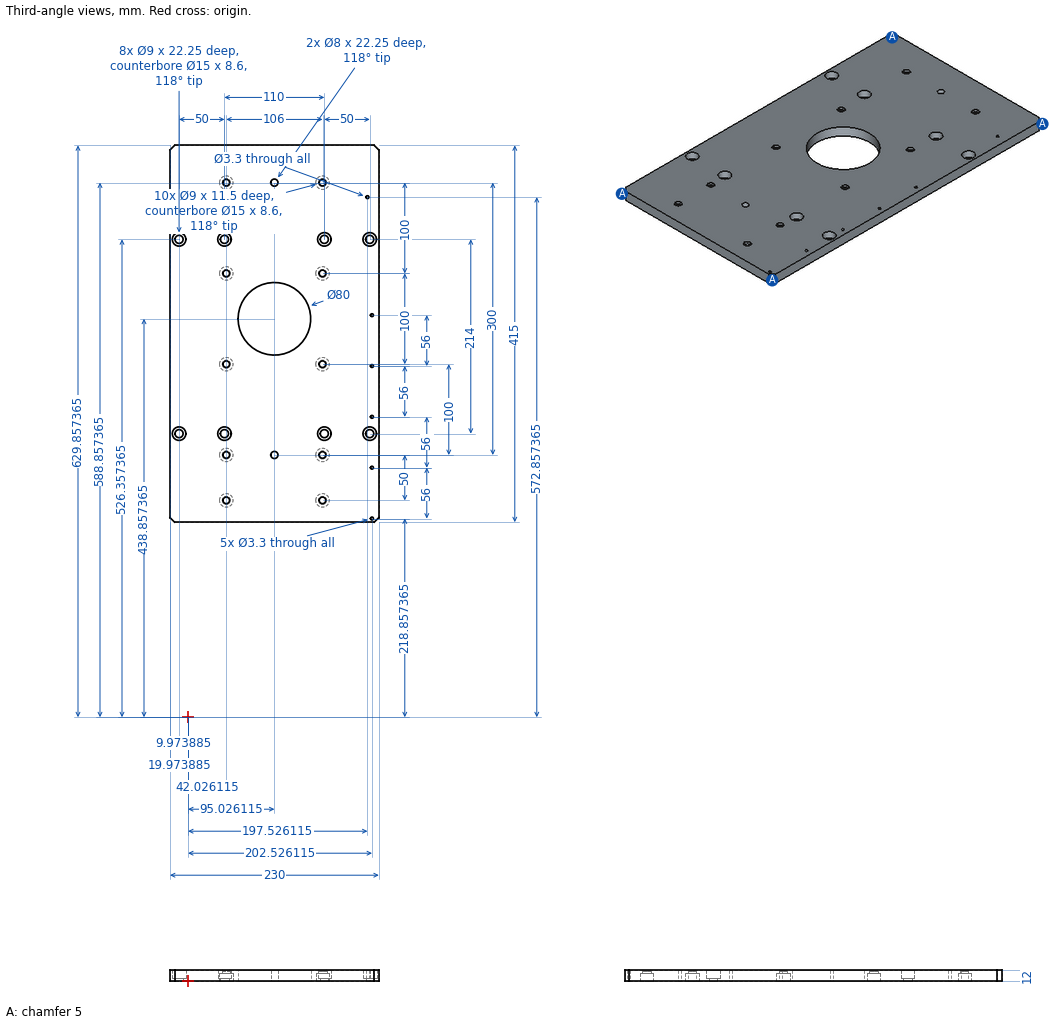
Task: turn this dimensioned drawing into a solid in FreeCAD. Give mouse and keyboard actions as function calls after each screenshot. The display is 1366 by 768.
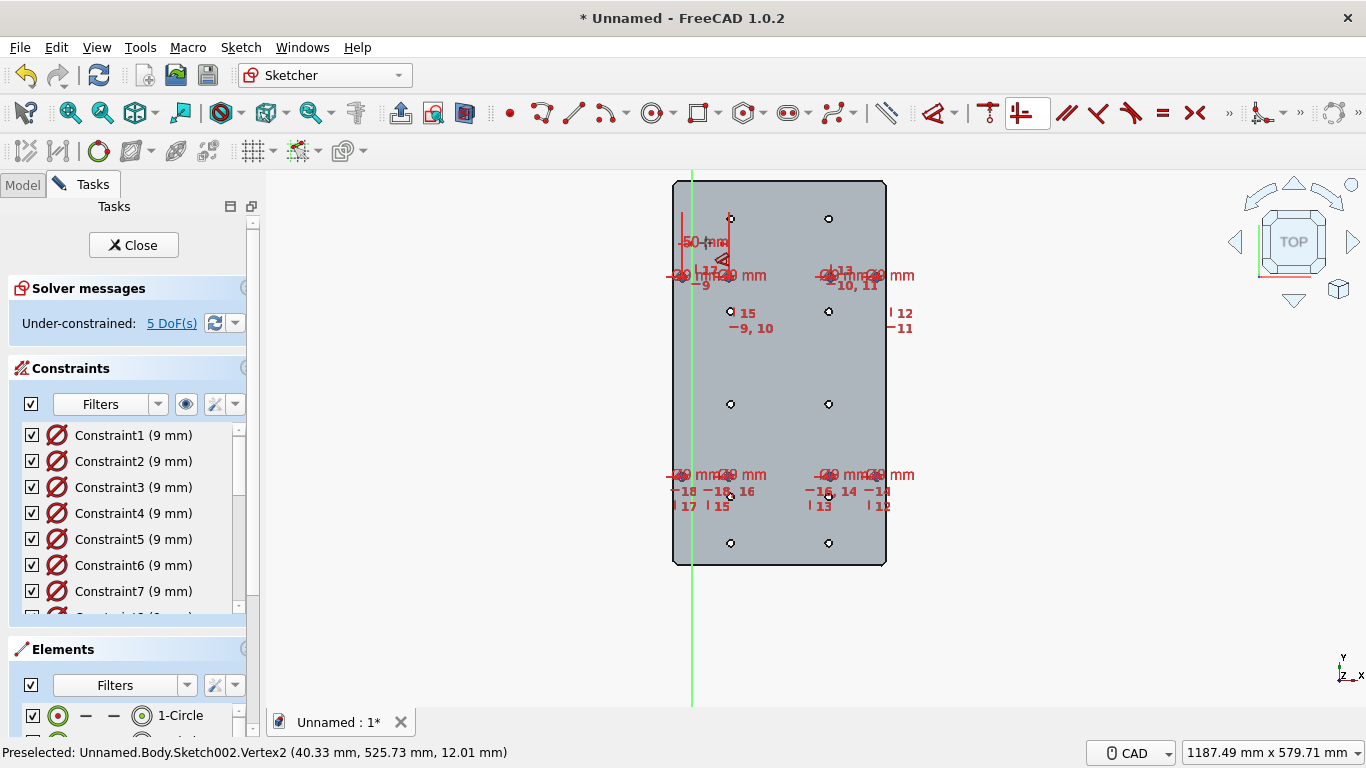
click(831, 277)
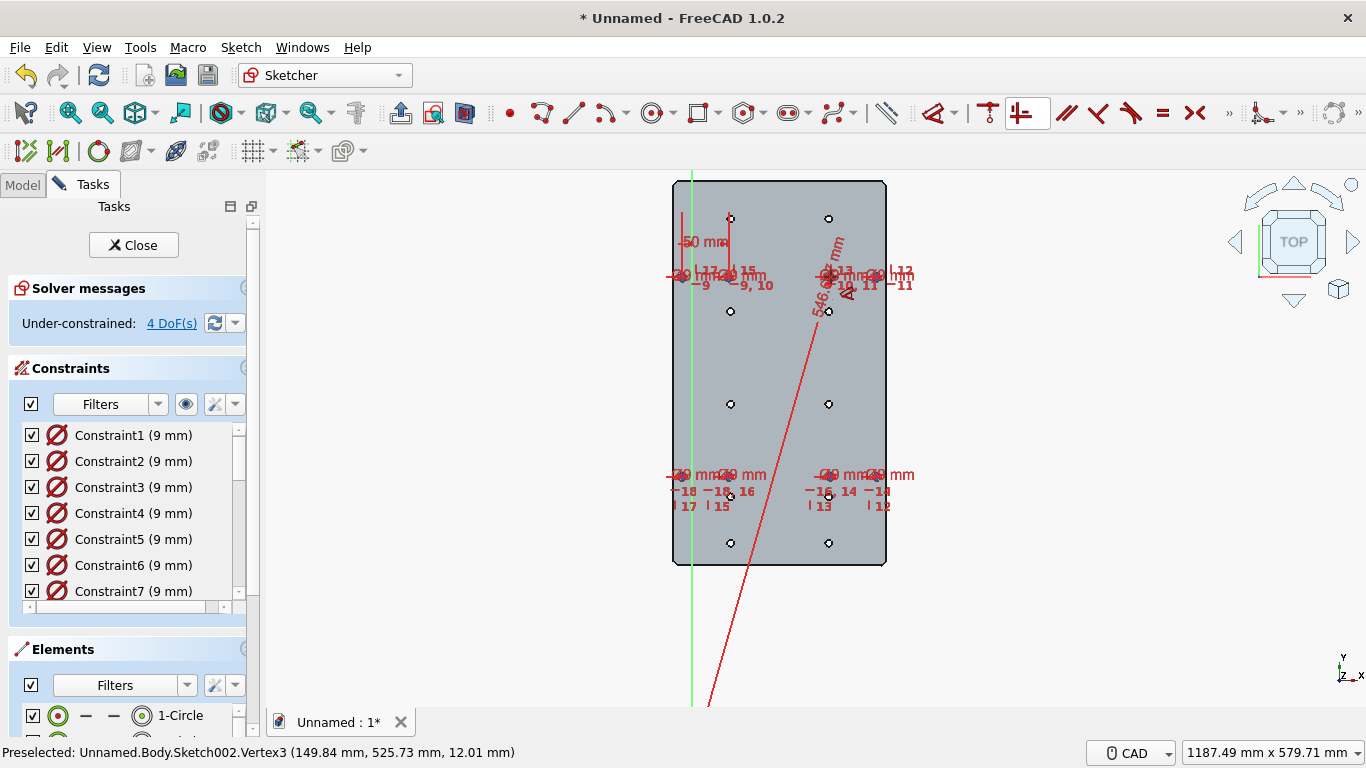
click(877, 277)
click(854, 243)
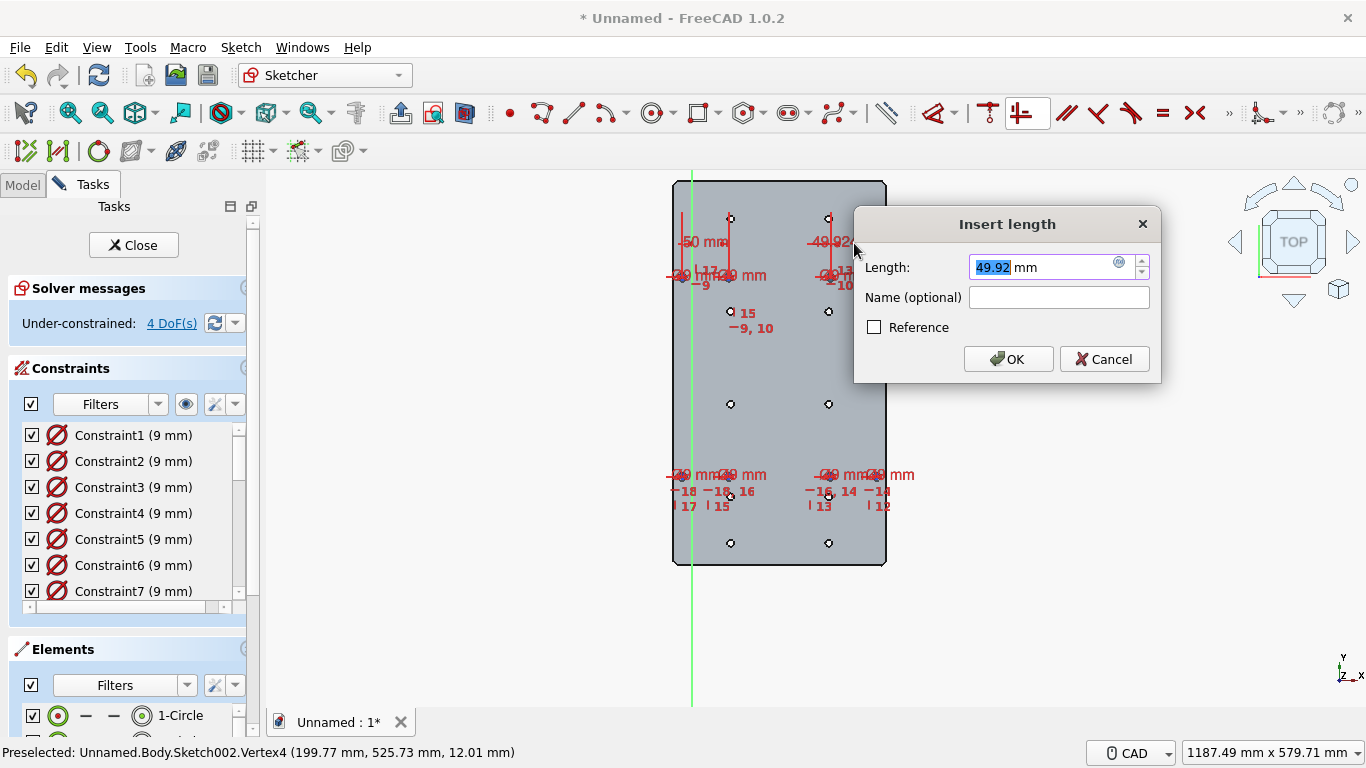
text(50)
key(Return)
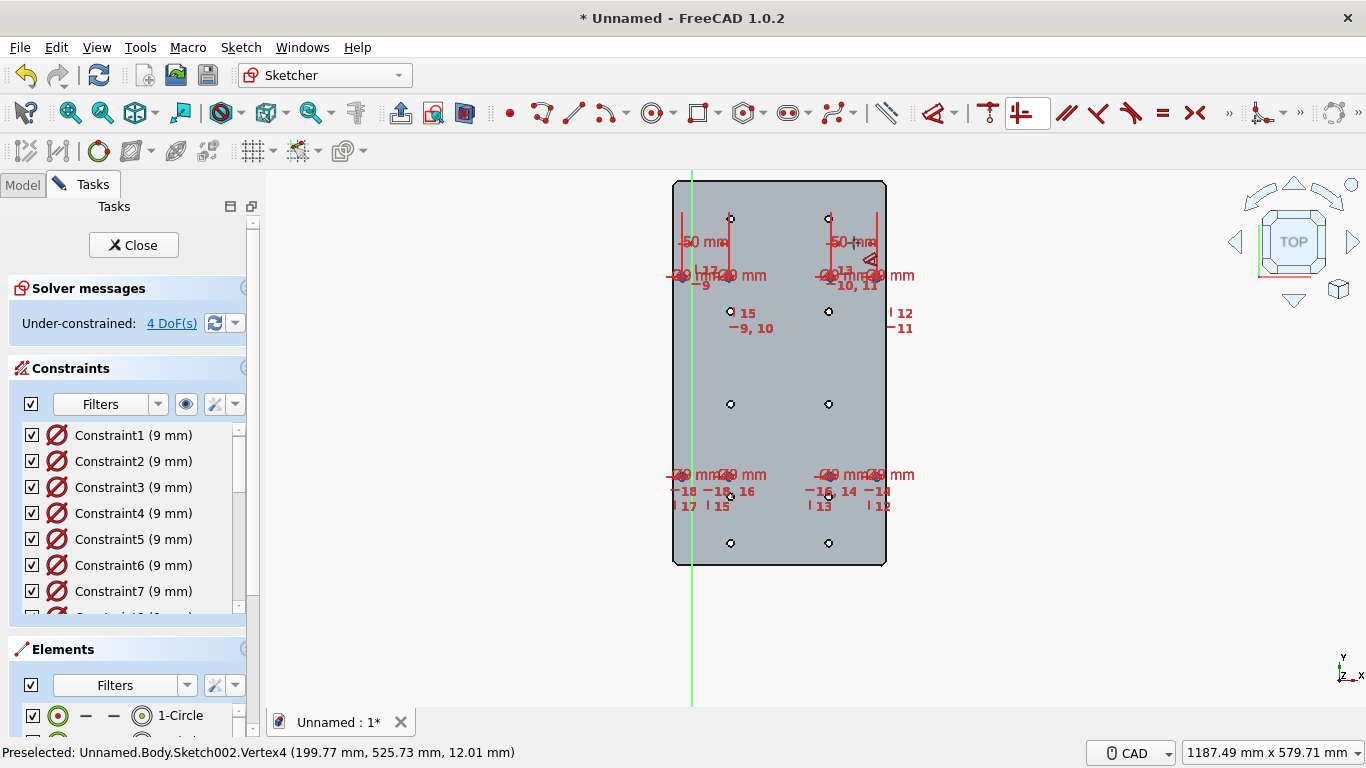
click(729, 277)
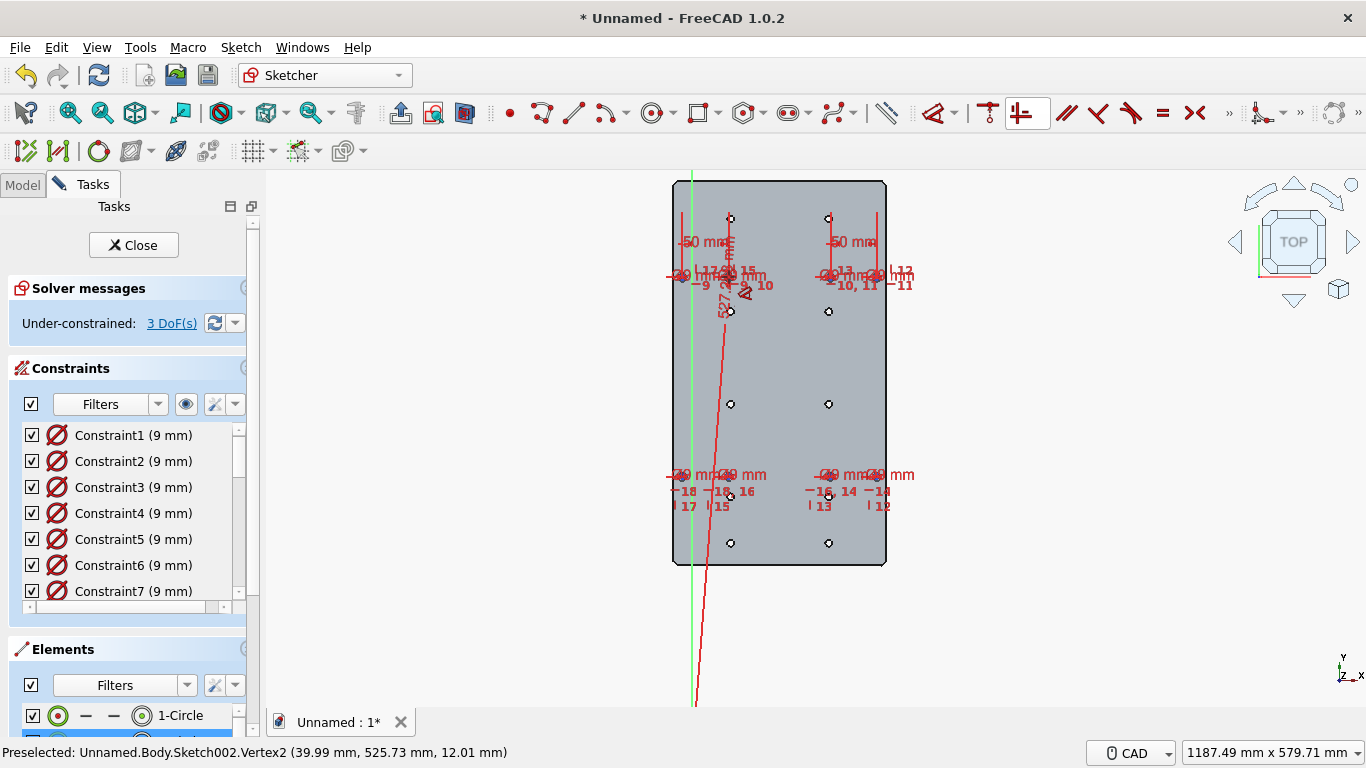
click(831, 277)
click(780, 243)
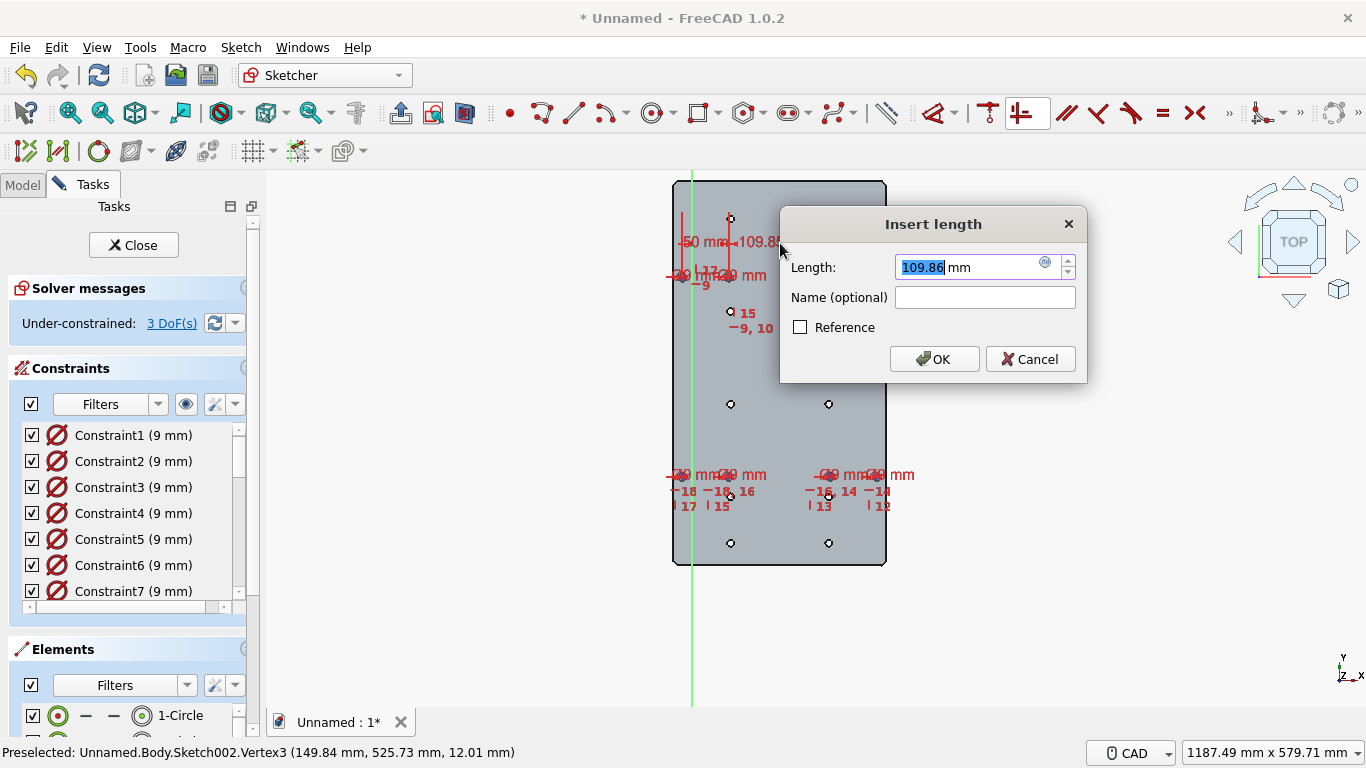
text(110)
key(Return)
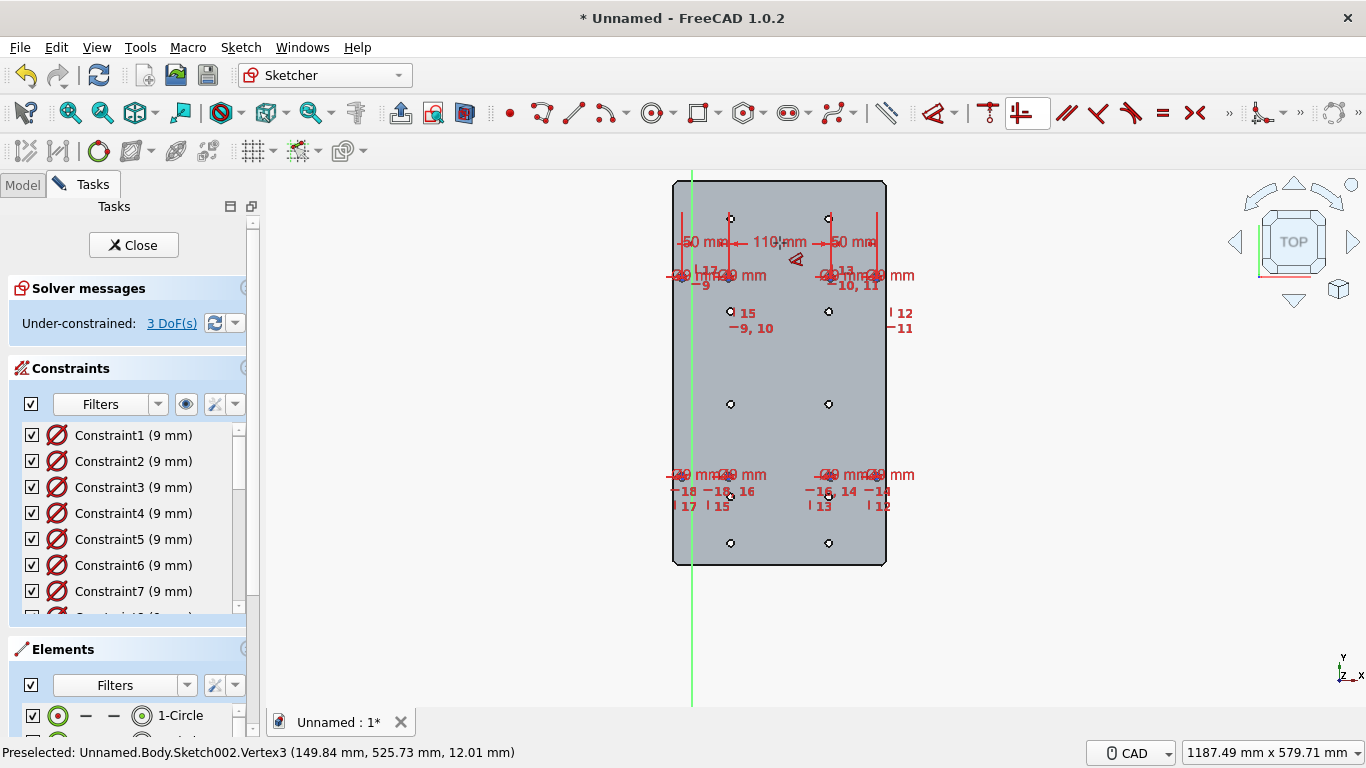
click(877, 277)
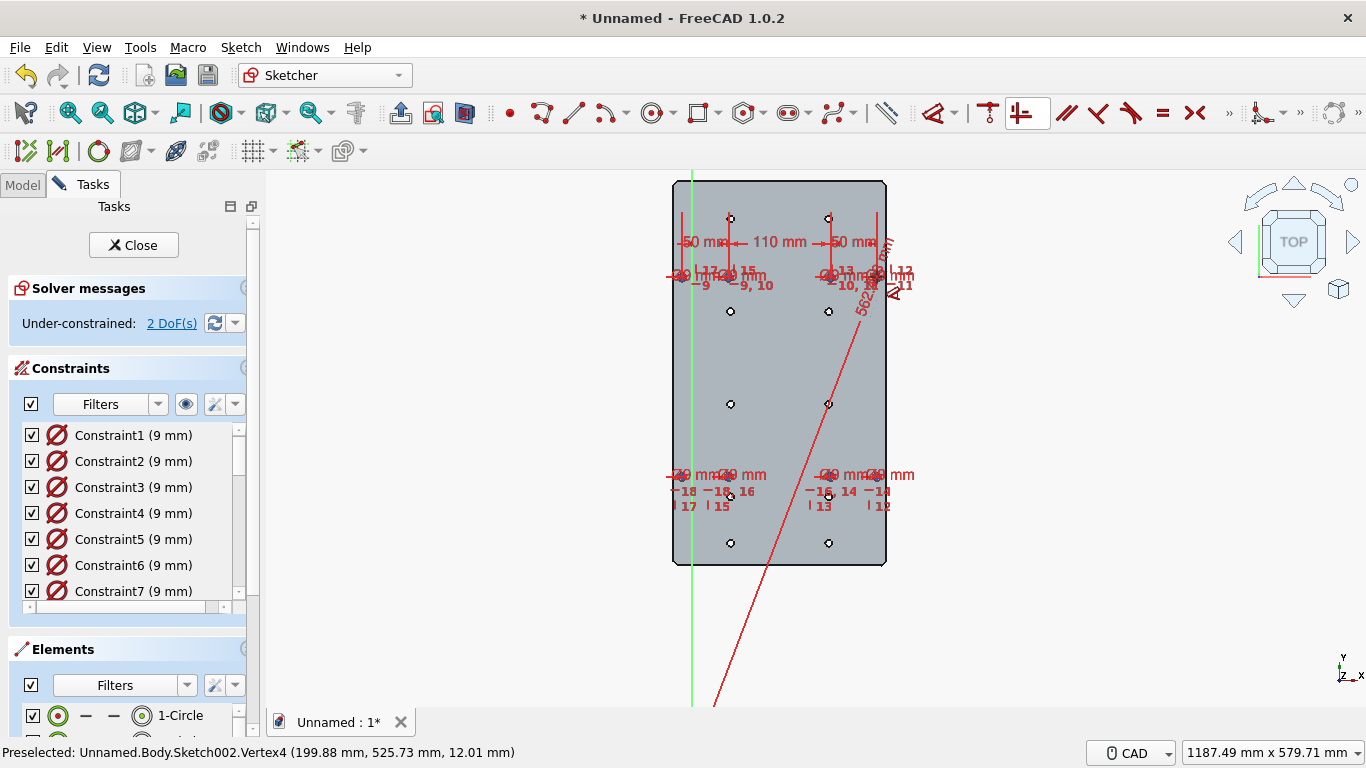
click(877, 477)
click(911, 377)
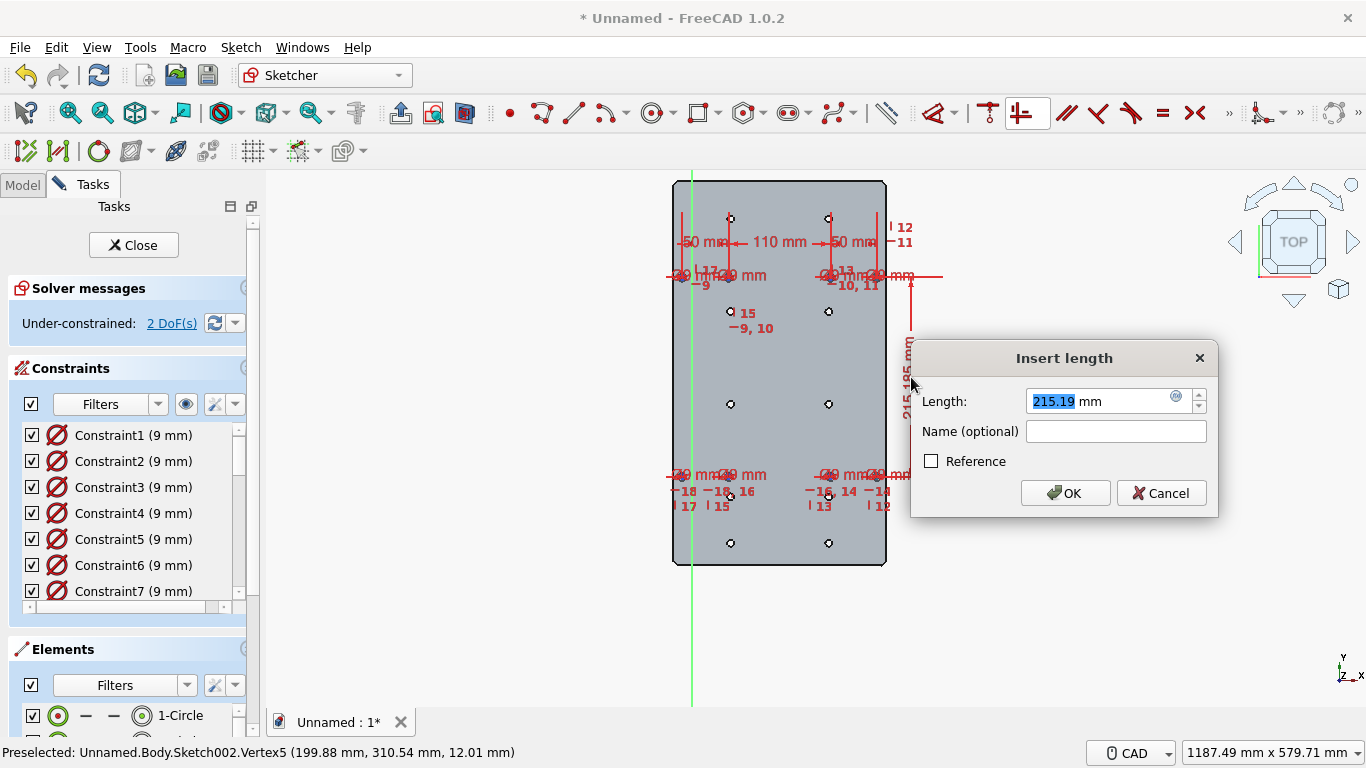
text(214)
key(Return)